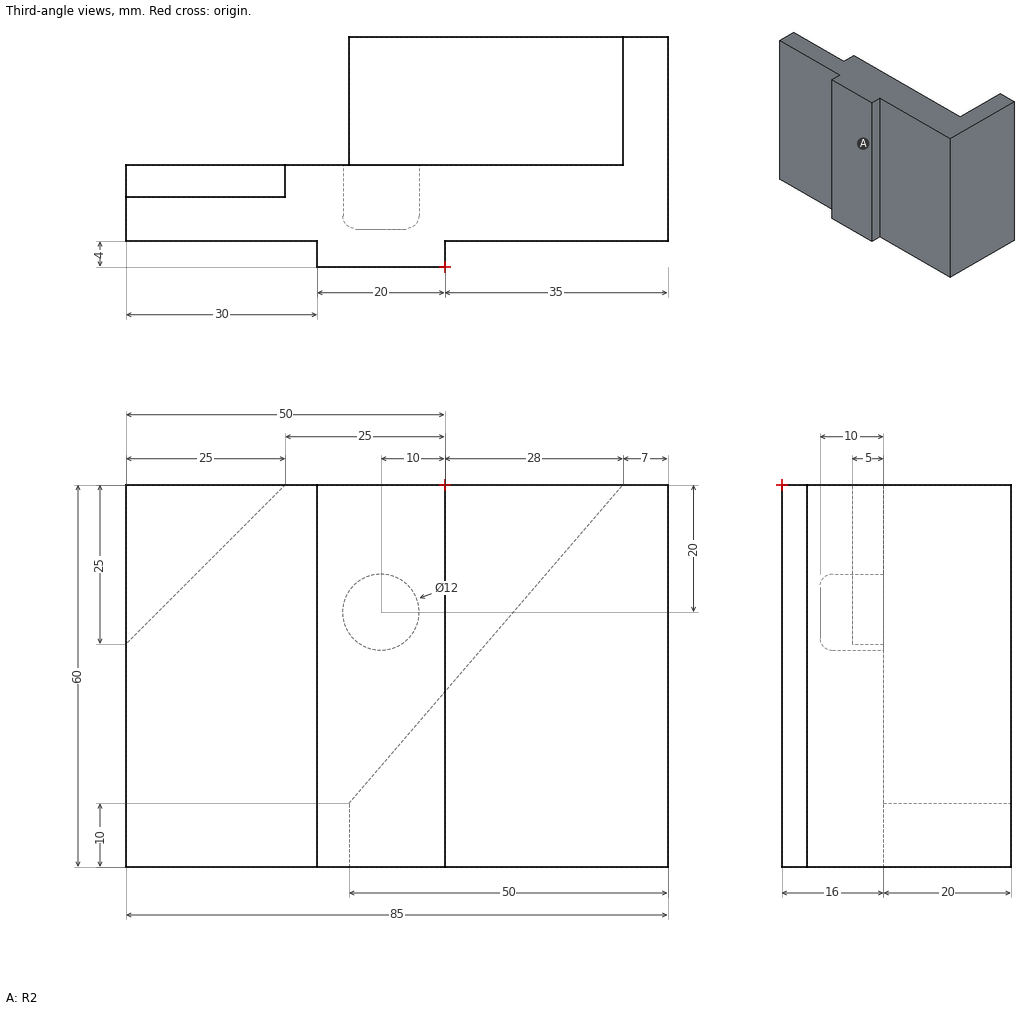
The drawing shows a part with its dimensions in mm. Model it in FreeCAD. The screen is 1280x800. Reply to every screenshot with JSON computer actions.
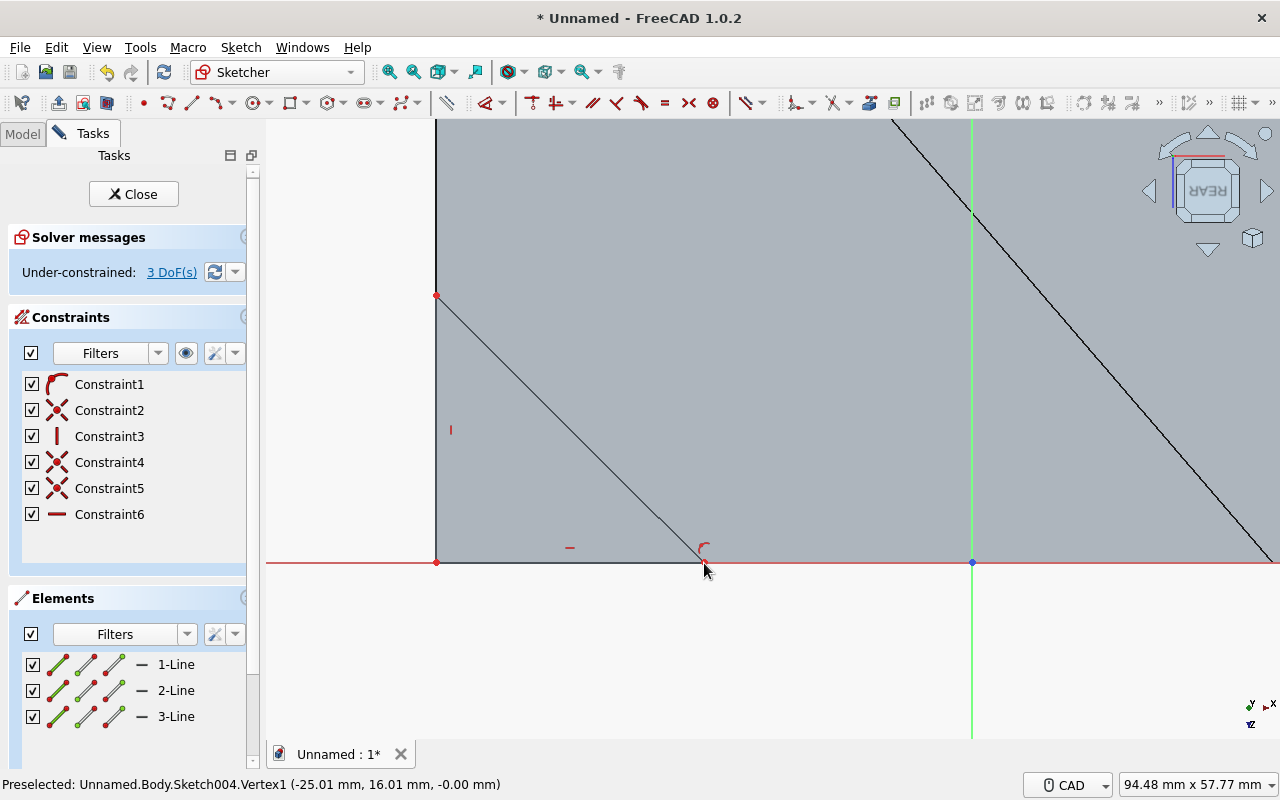
{"action": "left_click", "coordinate": [486, 104]}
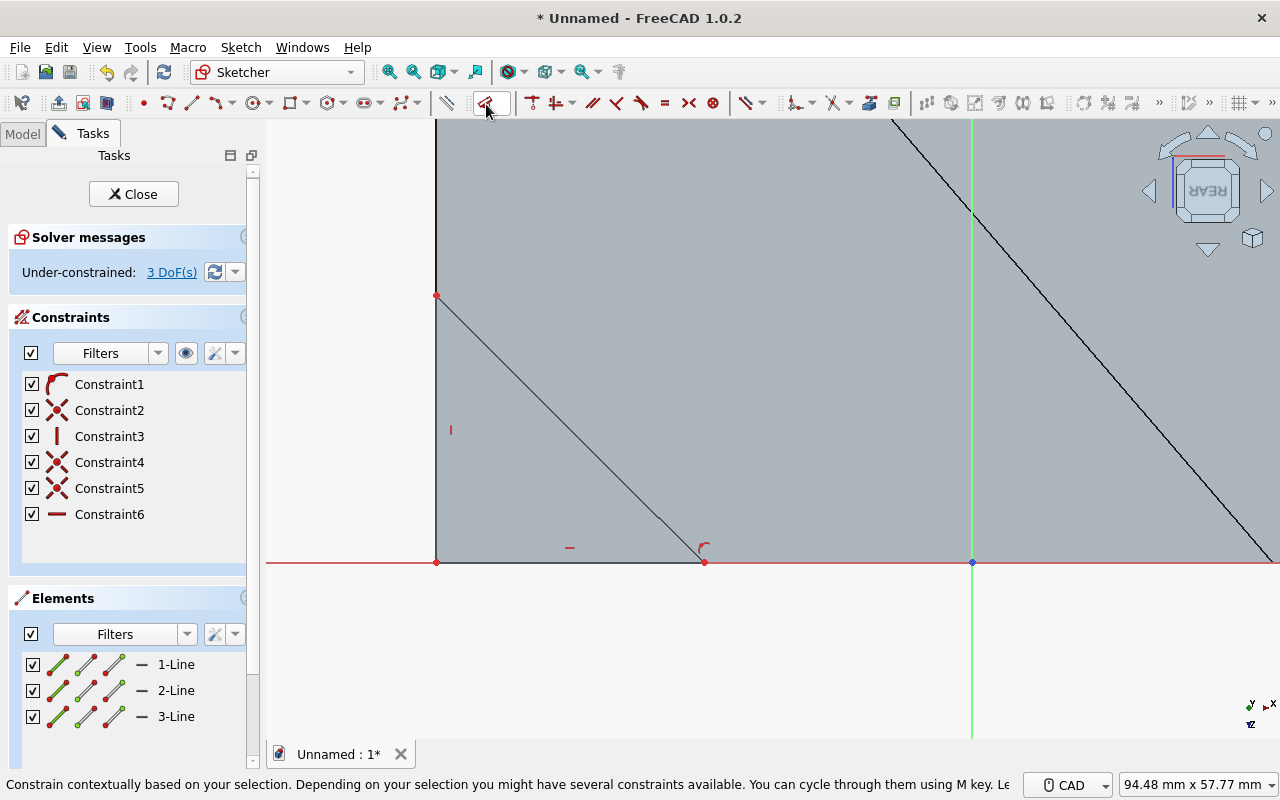
{"action": "left_click", "coordinate": [436, 376]}
{"action": "left_click", "coordinate": [402, 429]}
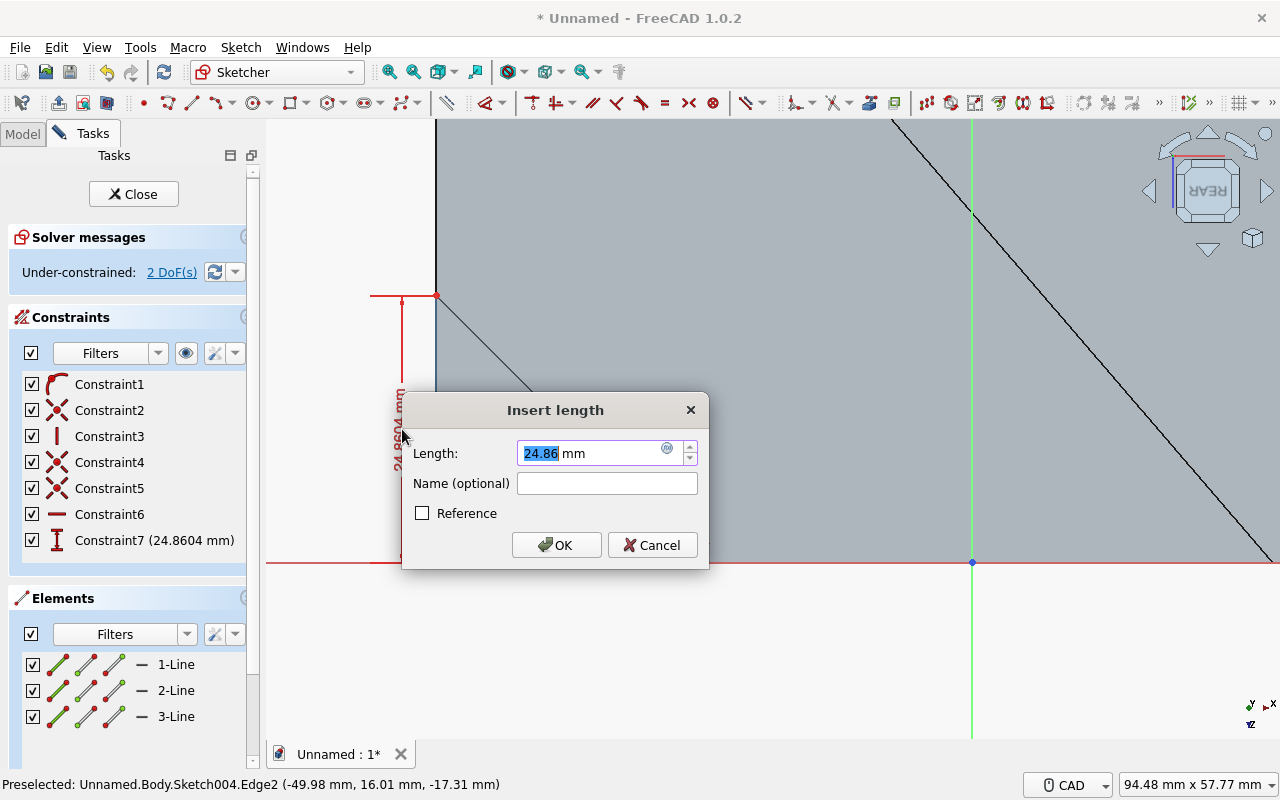
{"action": "type", "text": "25"}
{"action": "key", "text": "Return"}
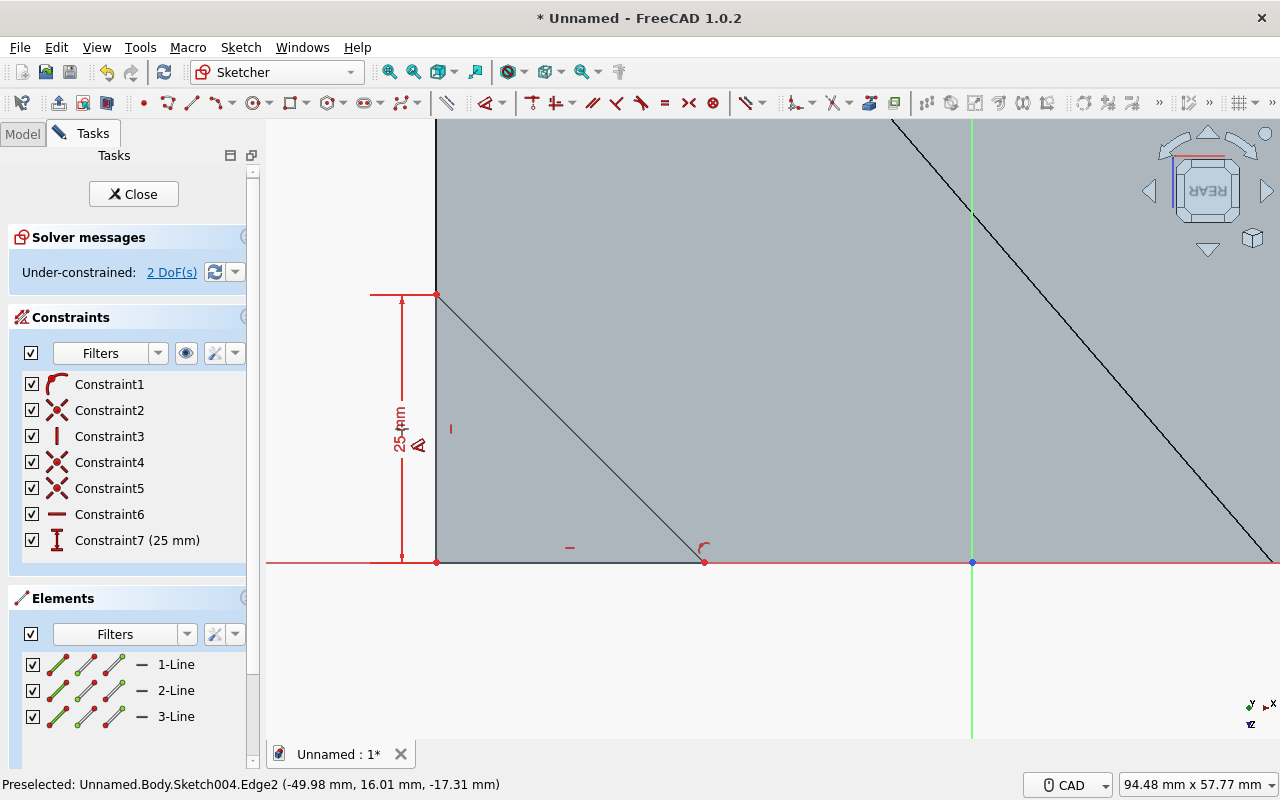
{"action": "left_click", "coordinate": [516, 563]}
{"action": "left_click", "coordinate": [570, 597]}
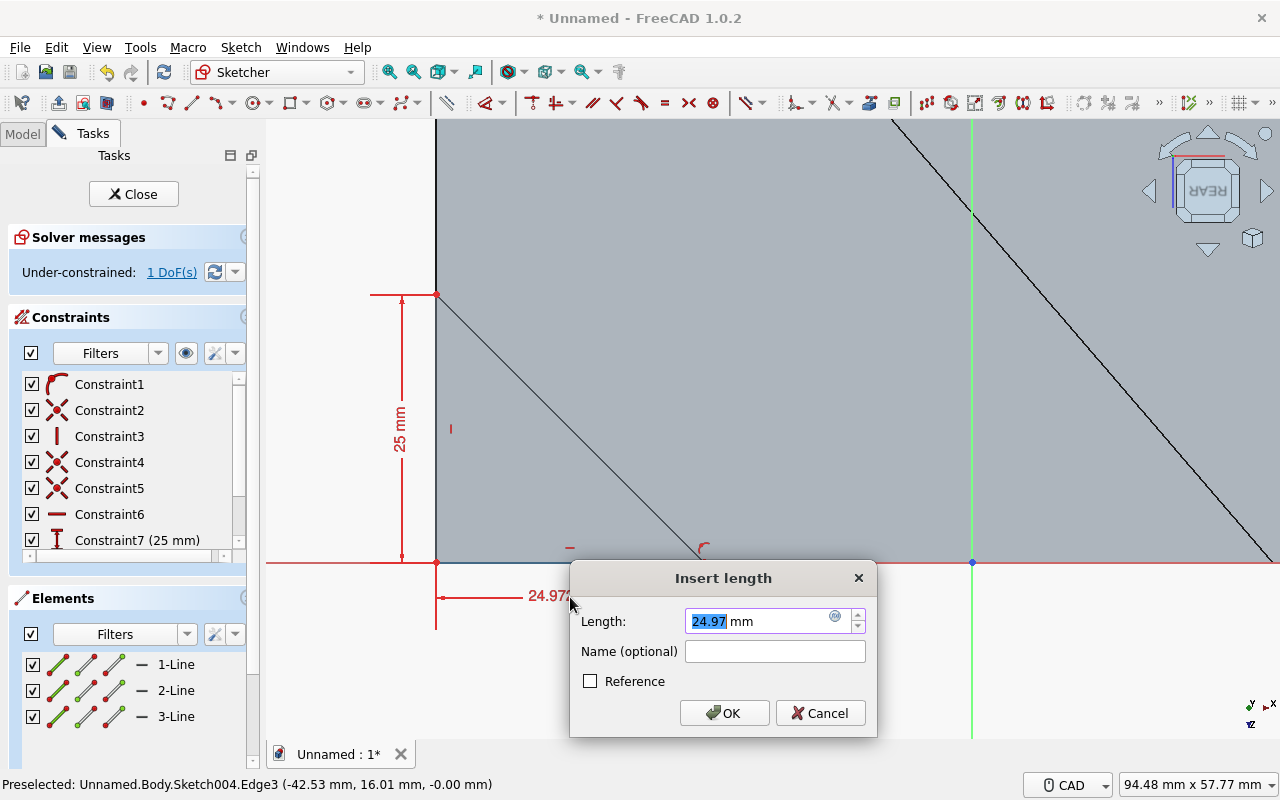
{"action": "type", "text": "25"}
{"action": "key", "text": "Return"}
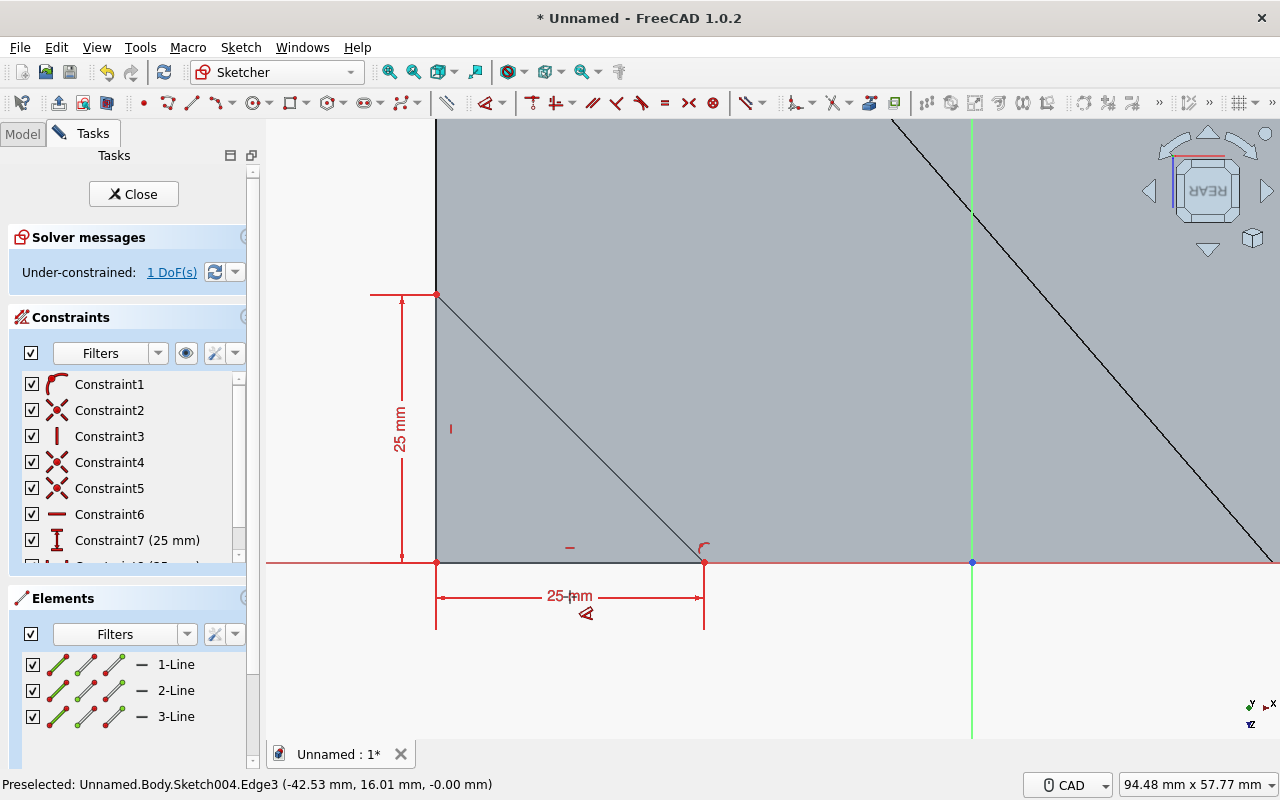
{"action": "left_click", "coordinate": [704, 563]}
{"action": "left_click", "coordinate": [838, 597]}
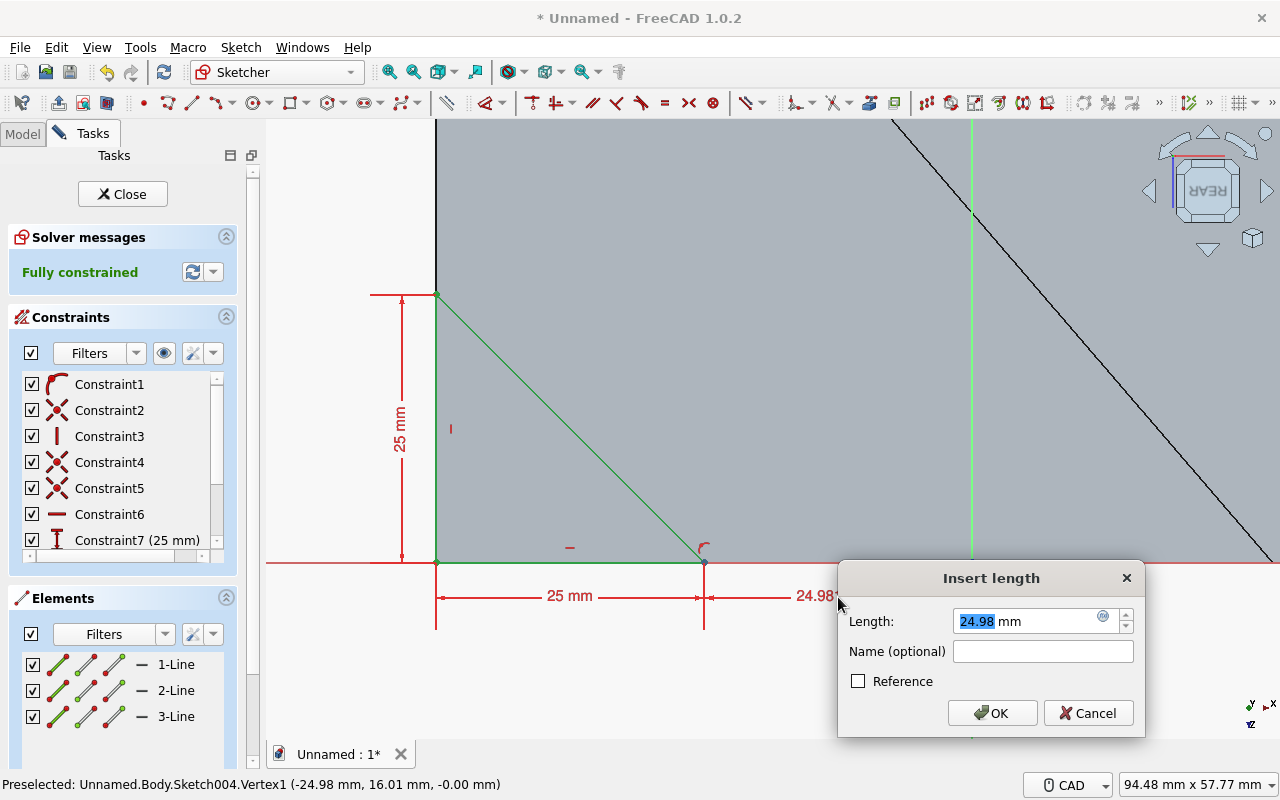
{"action": "type", "text": "25"}
{"action": "key", "text": "Return"}
{"action": "key", "text": "Escape"}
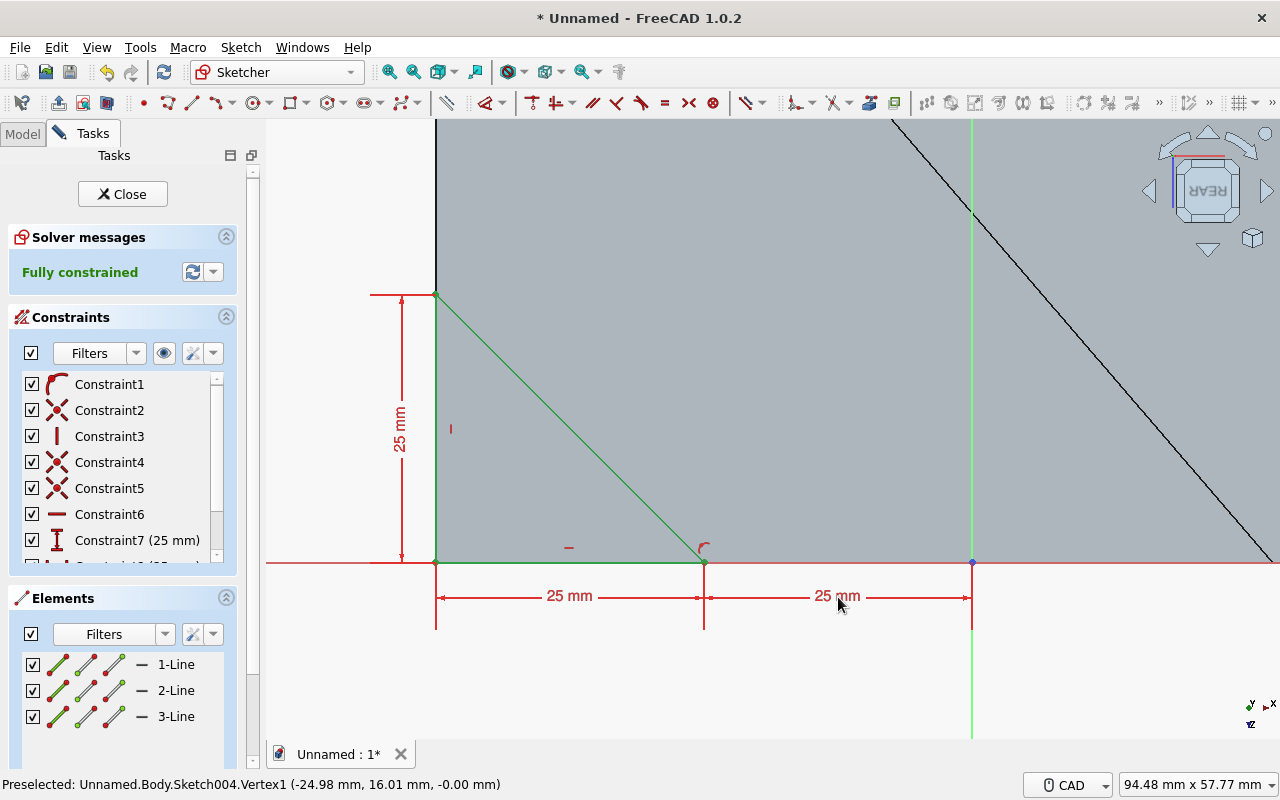
{"action": "left_click", "coordinate": [123, 194]}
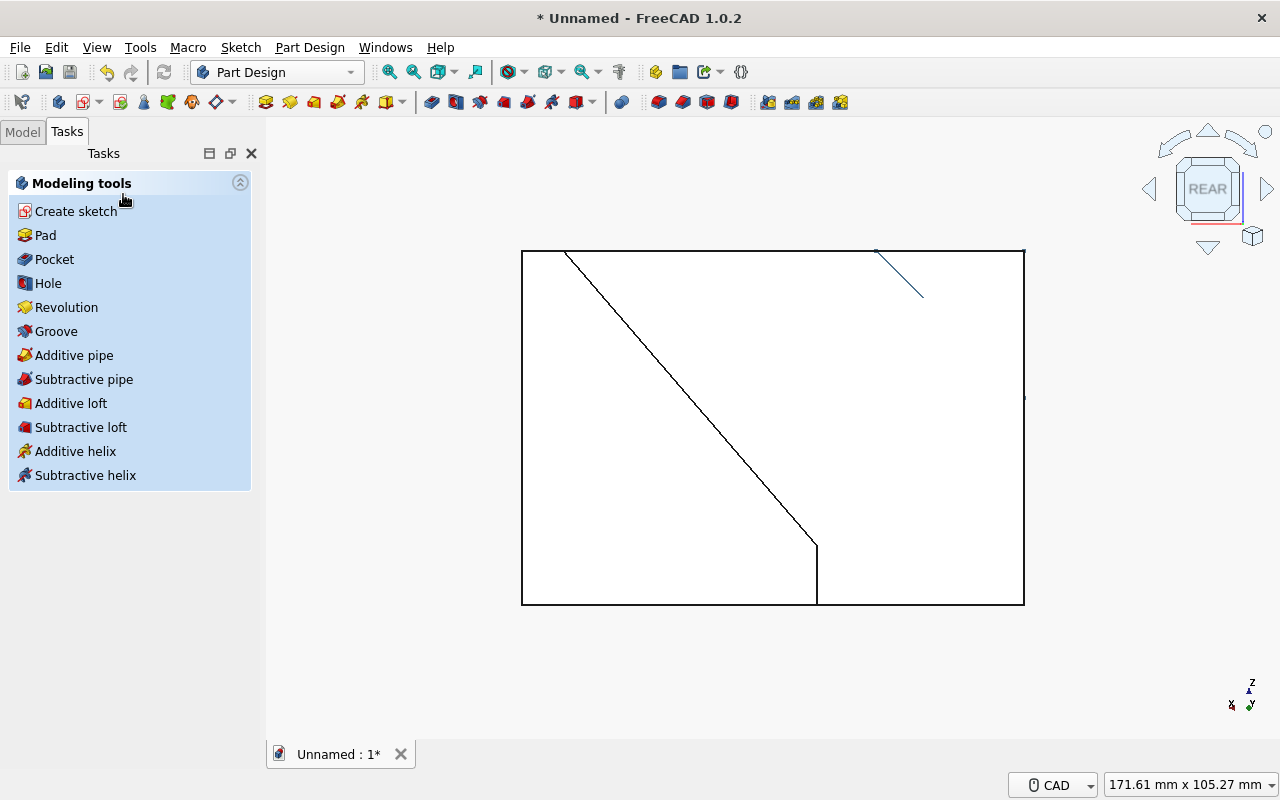
{"action": "left_click", "coordinate": [432, 102]}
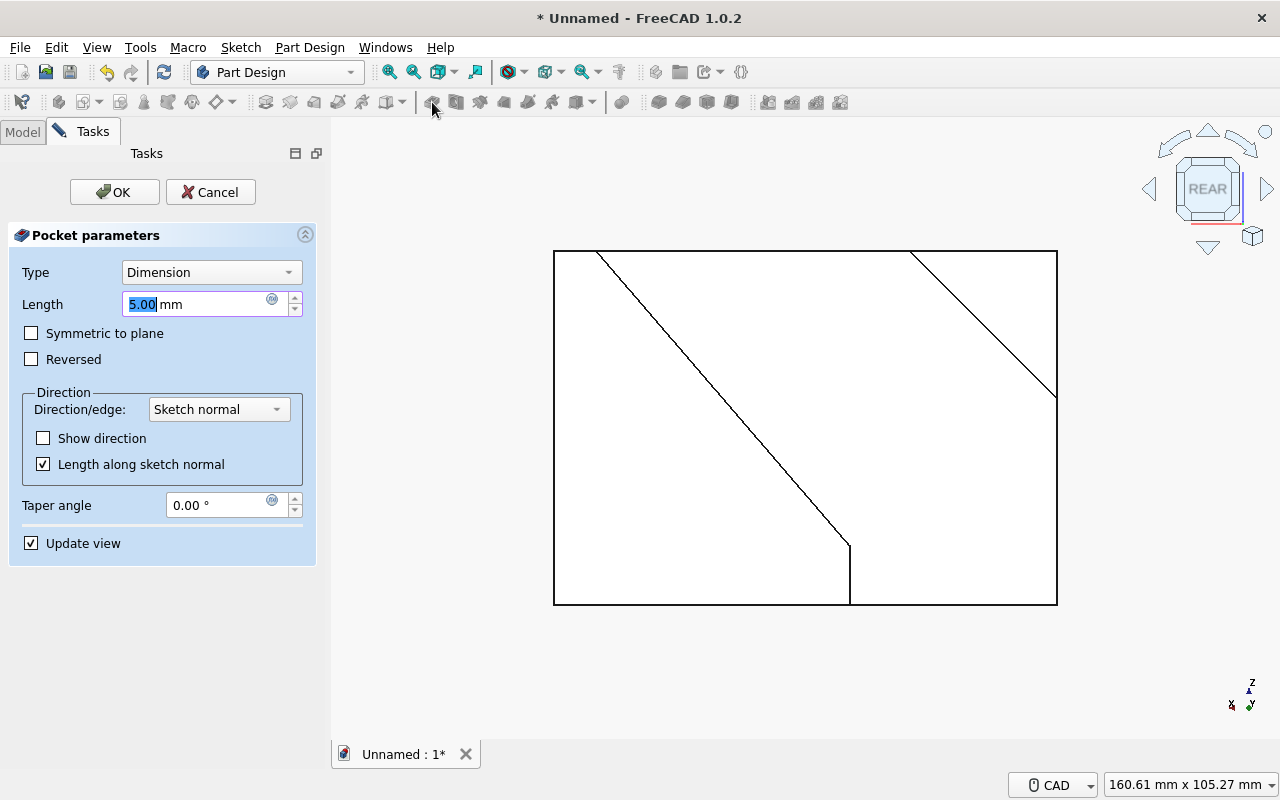
{"action": "type", "text": "5"}
{"action": "key", "text": "Tab"}